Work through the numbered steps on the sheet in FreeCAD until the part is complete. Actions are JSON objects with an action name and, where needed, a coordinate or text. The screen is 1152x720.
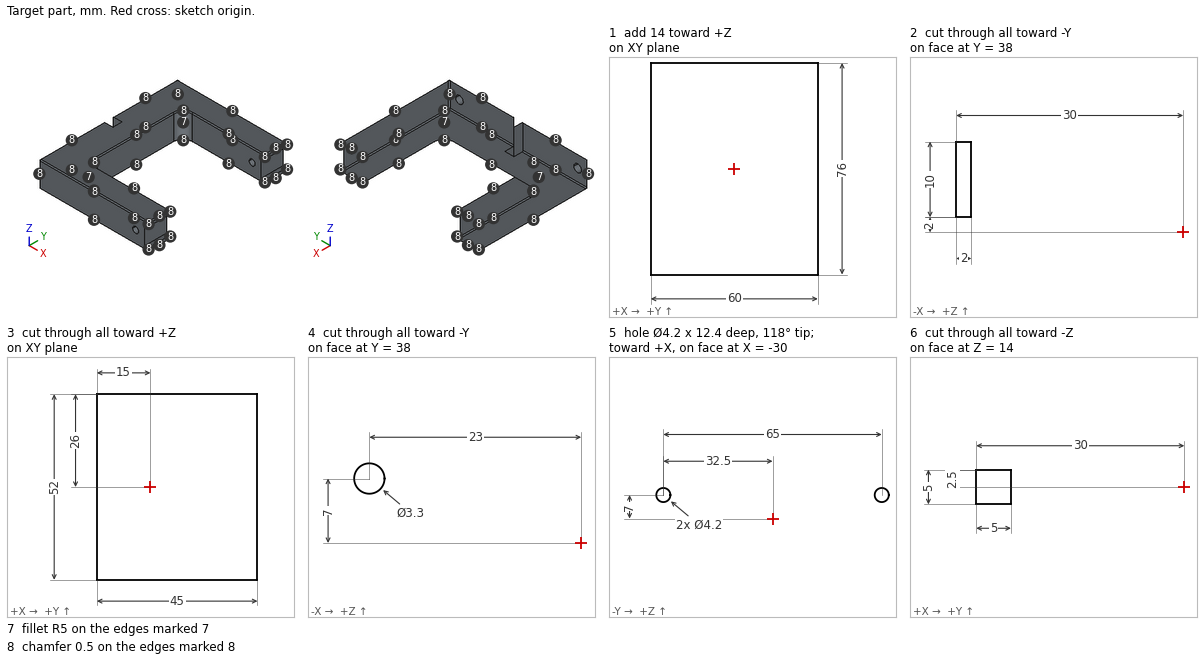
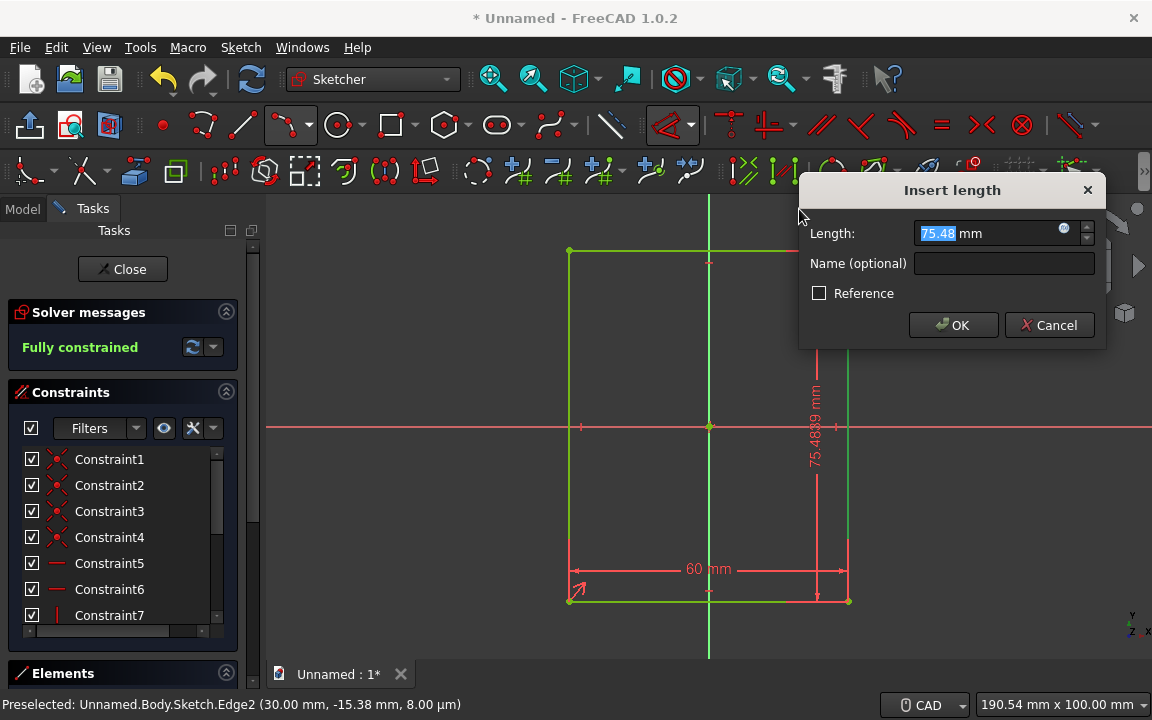
{"action": "type", "text": "76"}
{"action": "key", "text": "Return"}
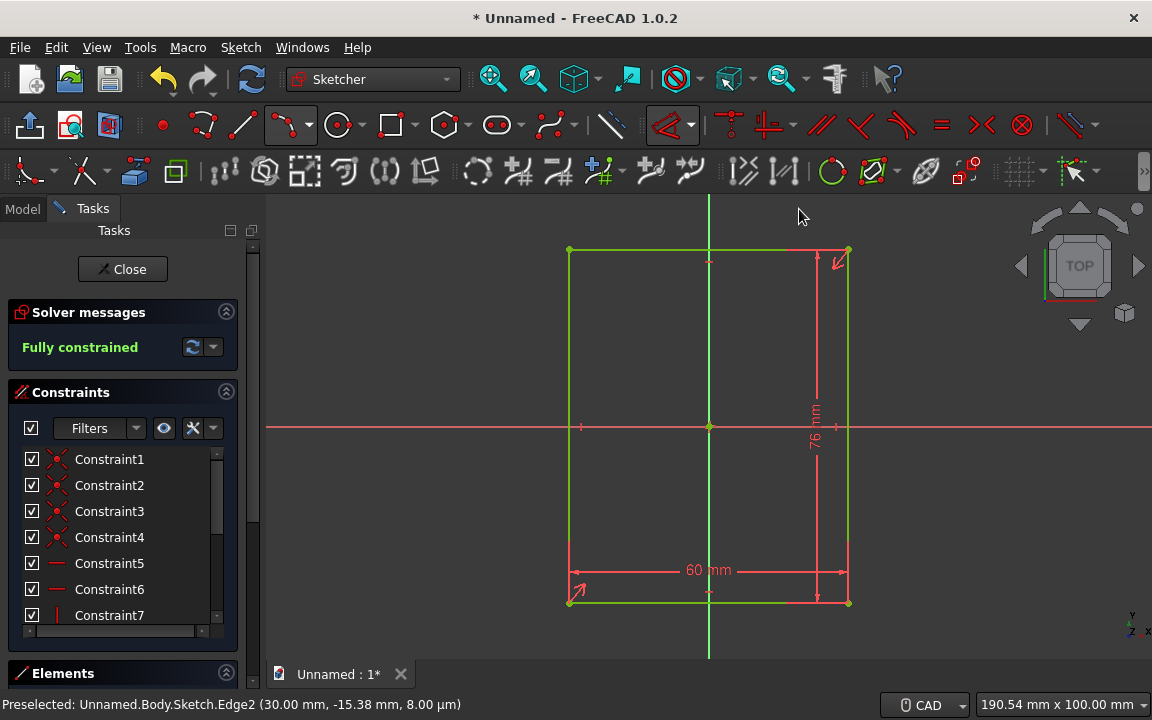
{"action": "left_click", "coordinate": [123, 269]}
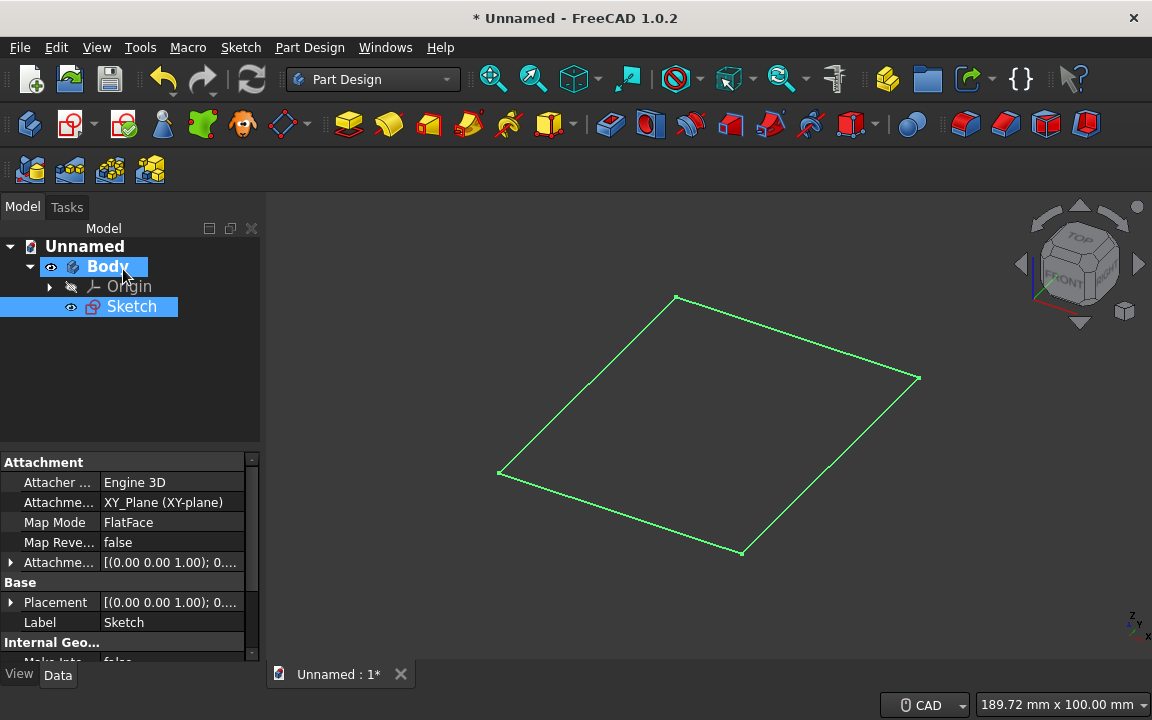
{"action": "left_click", "coordinate": [350, 124]}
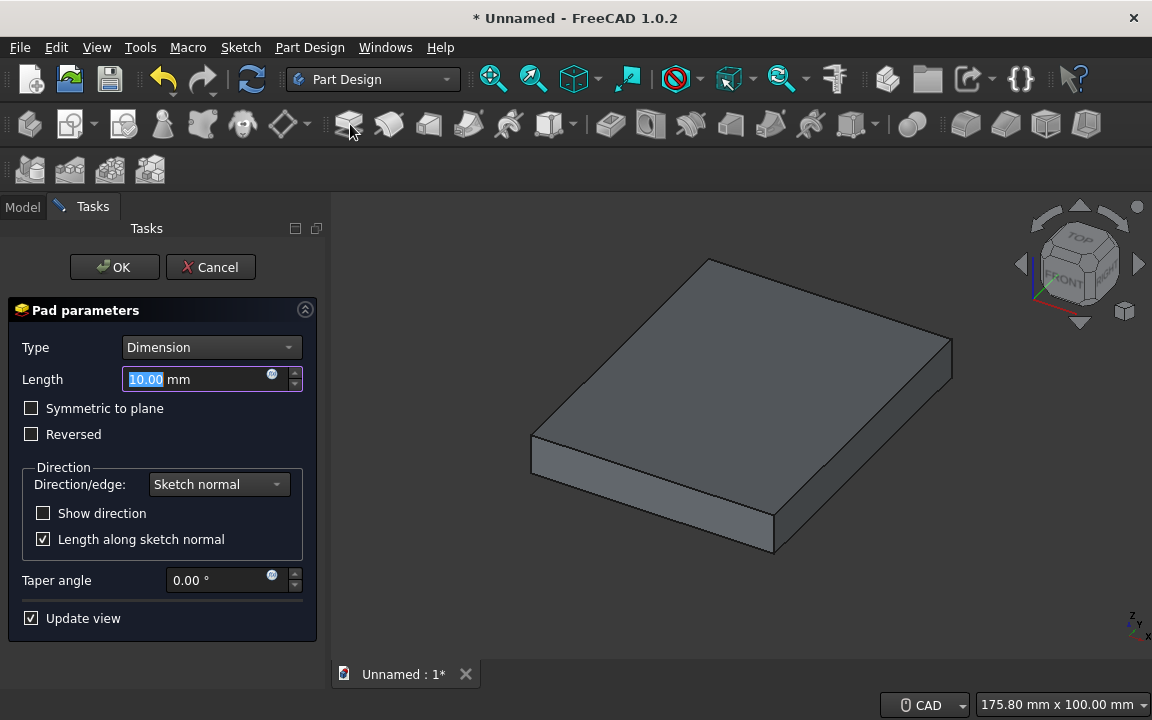
{"action": "type", "text": "14"}
{"action": "key", "text": "Tab"}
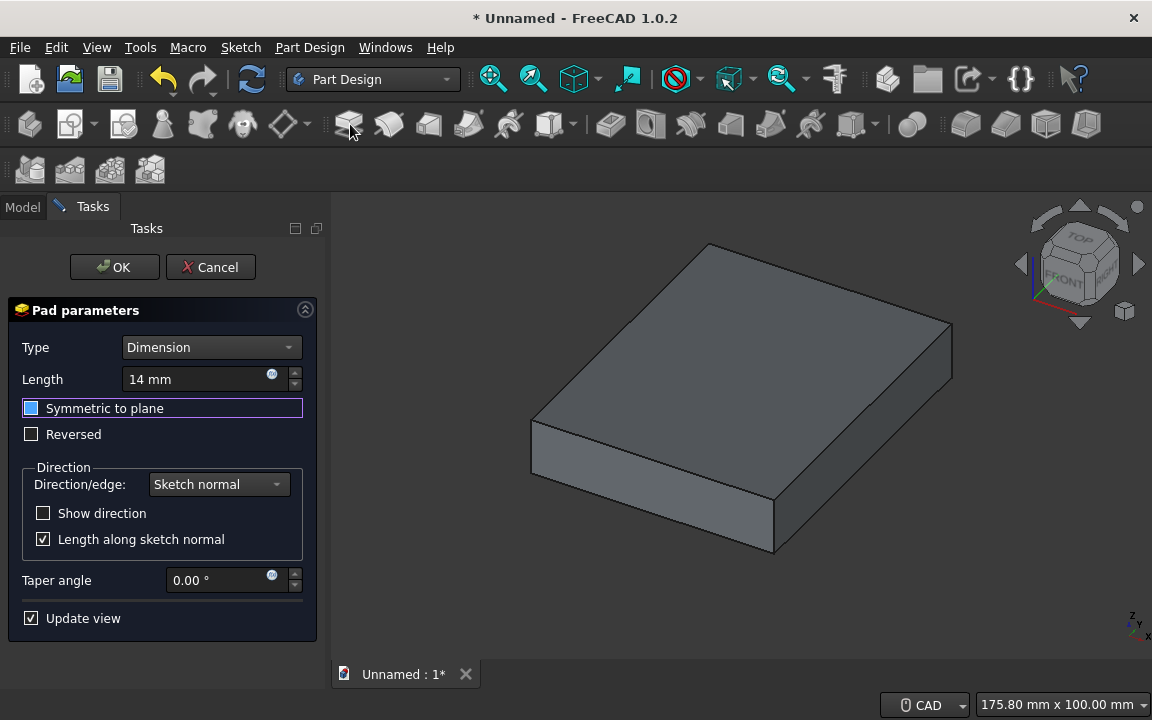
{"action": "left_click", "coordinate": [115, 267]}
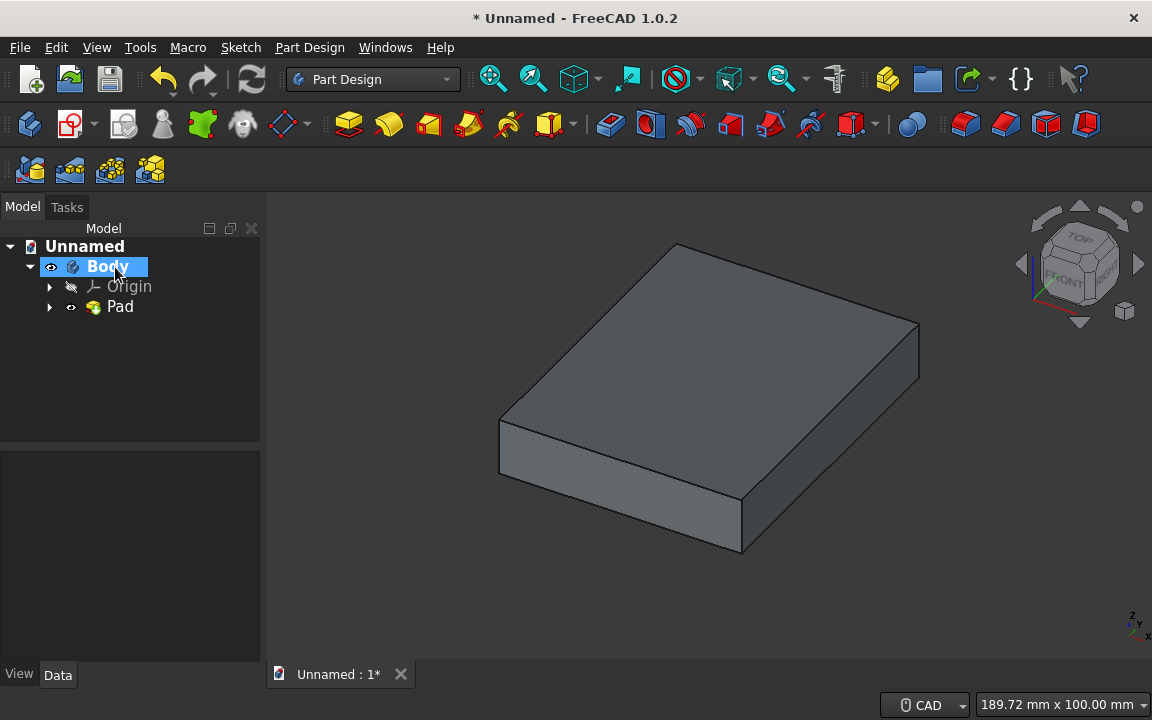
{"action": "key", "text": "4"}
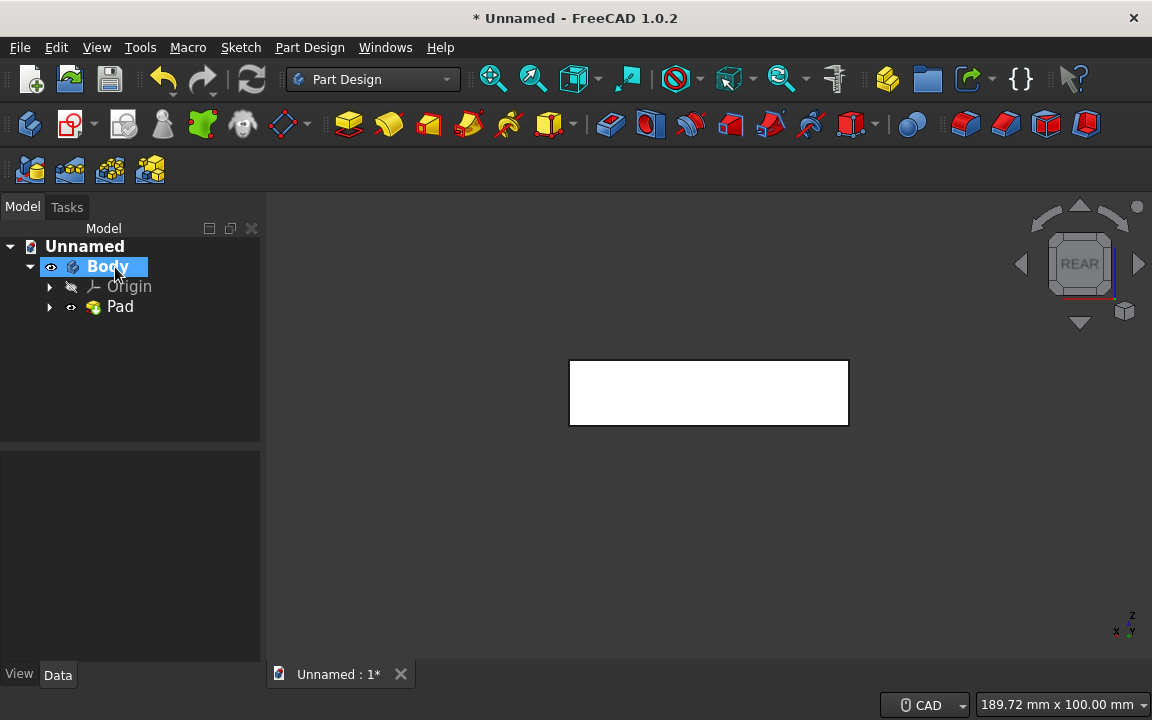
{"action": "key", "text": "v f"}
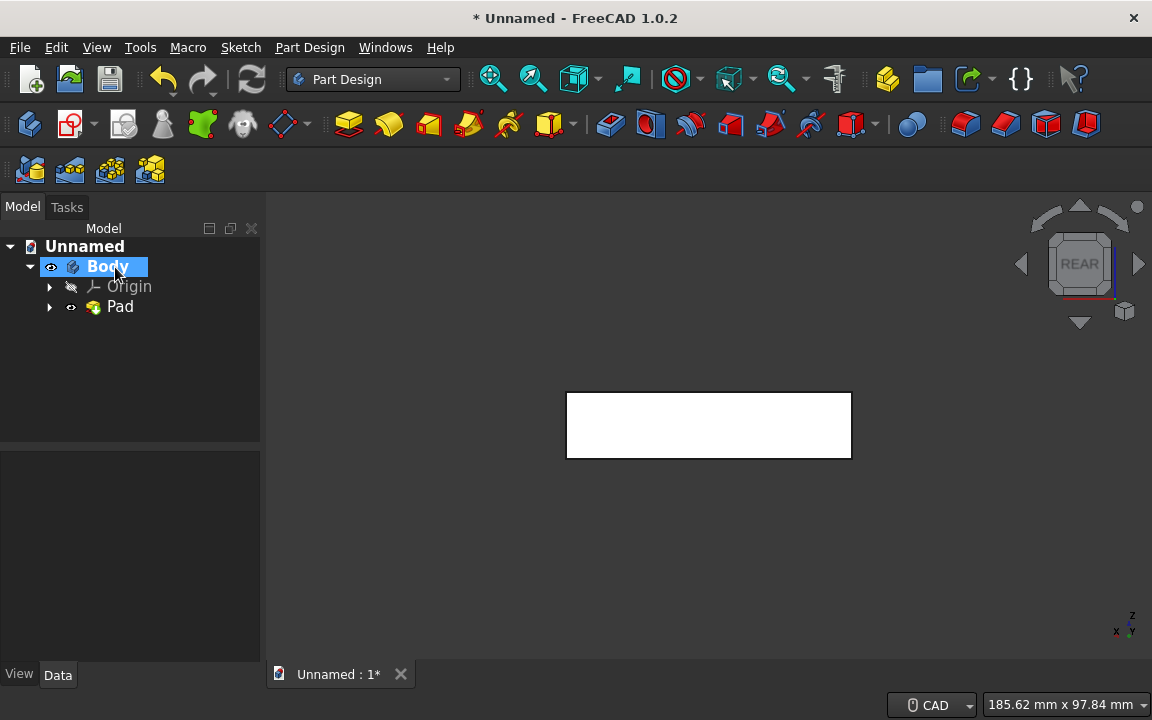
{"action": "left_click", "coordinate": [627, 425]}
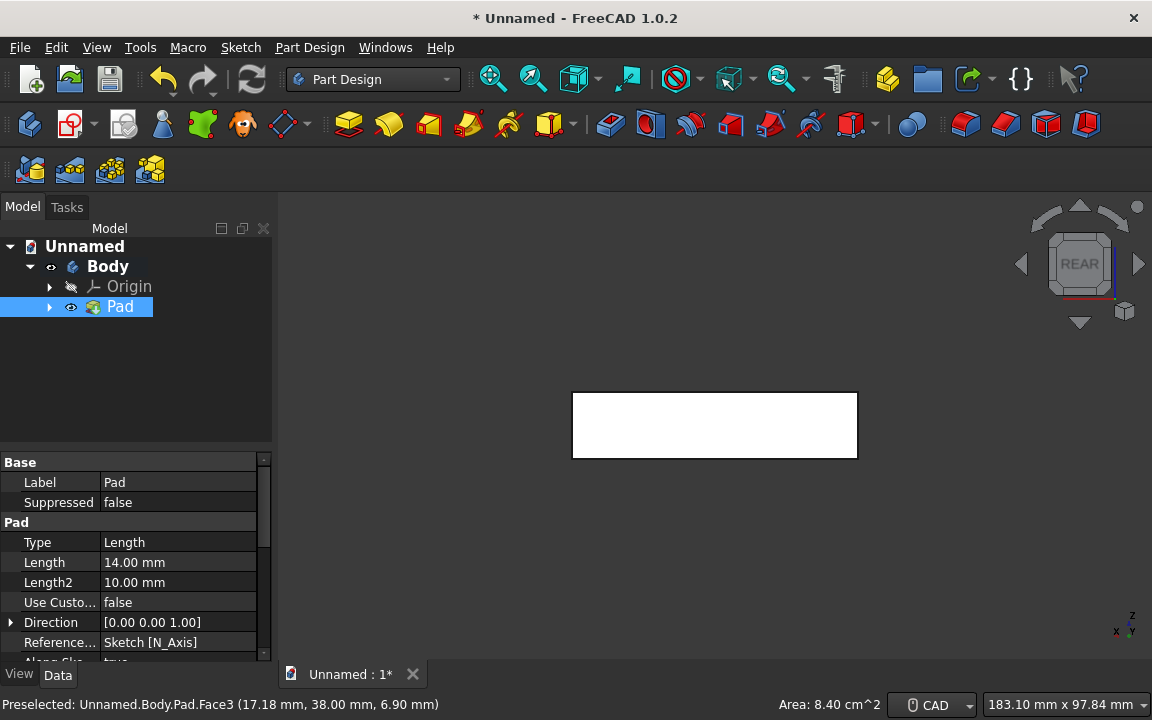
{"action": "left_click", "coordinate": [70, 124]}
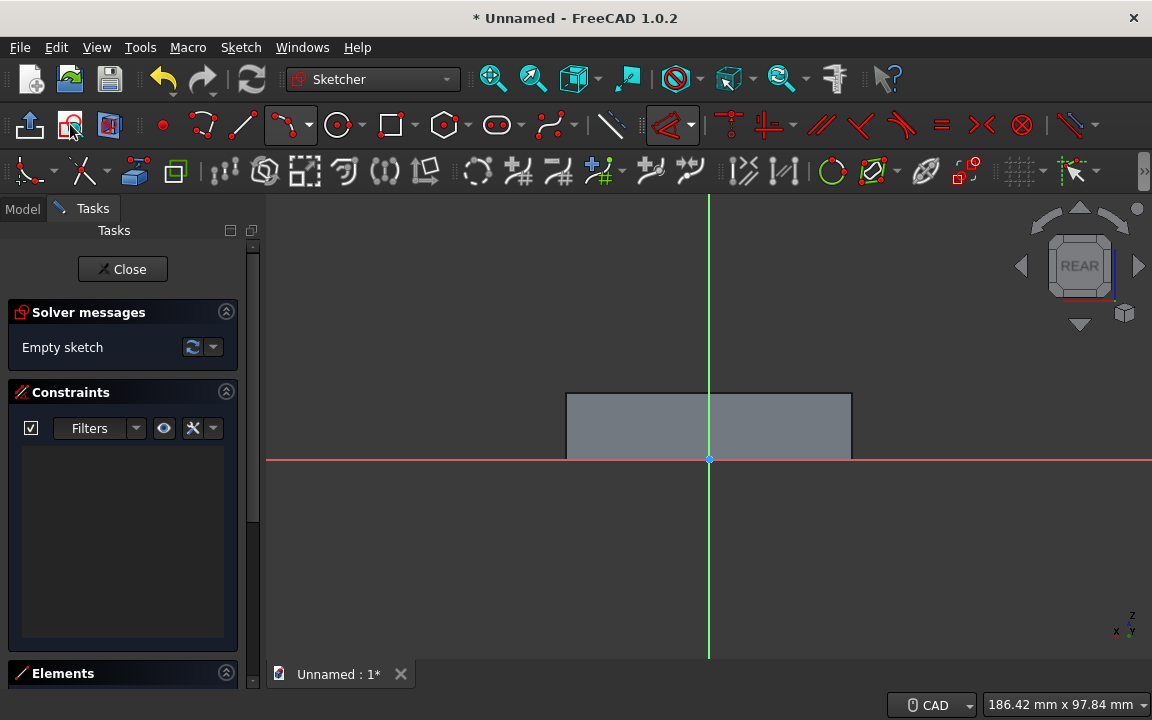
{"action": "scroll", "coordinate": [557, 426], "scroll_direction": "up", "scroll_amount": 9}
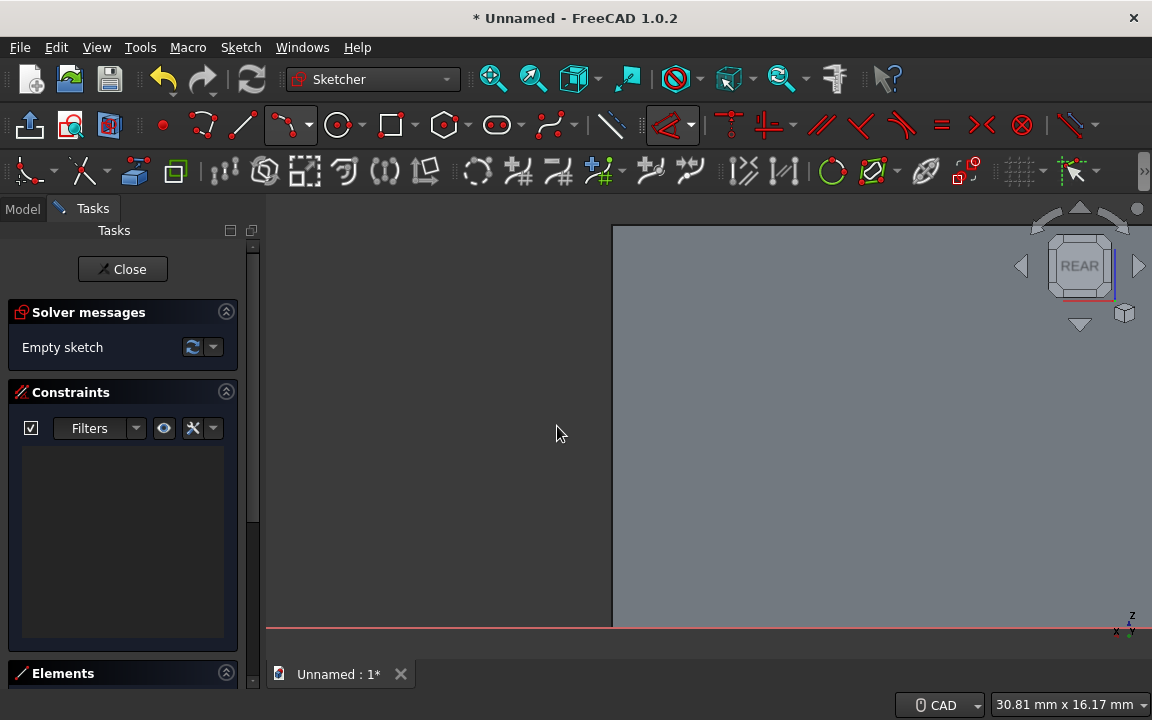
{"action": "key", "text": "g r"}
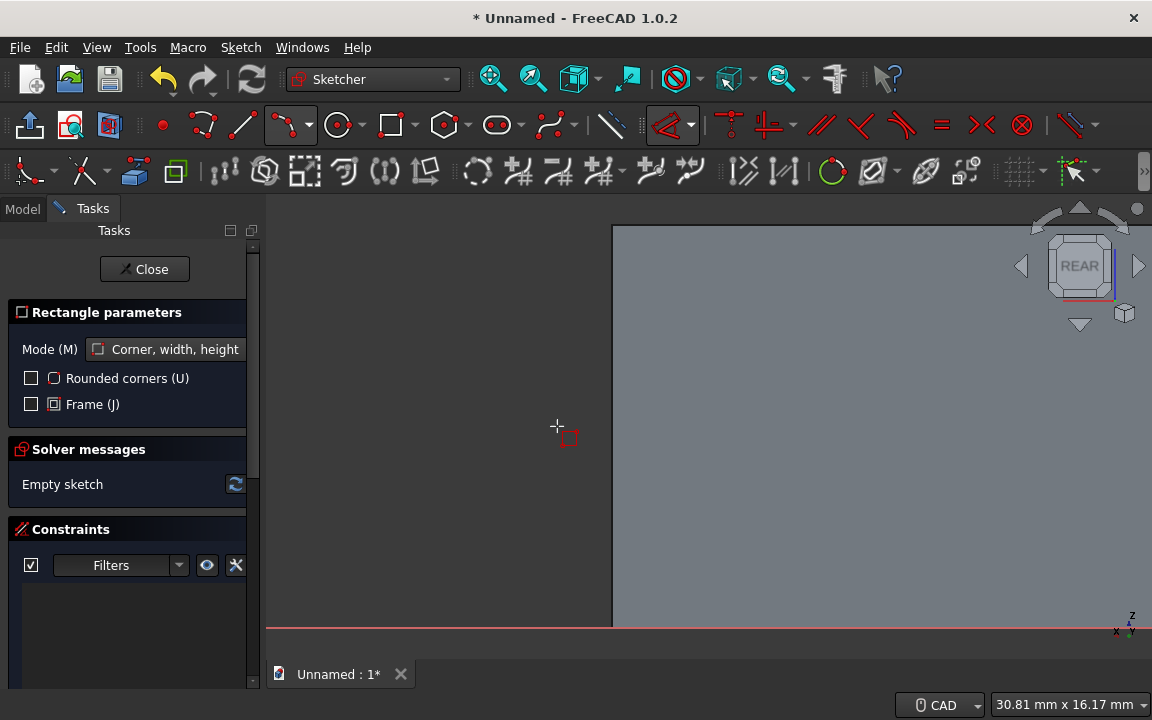
{"action": "left_click", "coordinate": [612, 283]}
{"action": "left_click", "coordinate": [670, 570]}
{"action": "key", "text": "Escape"}